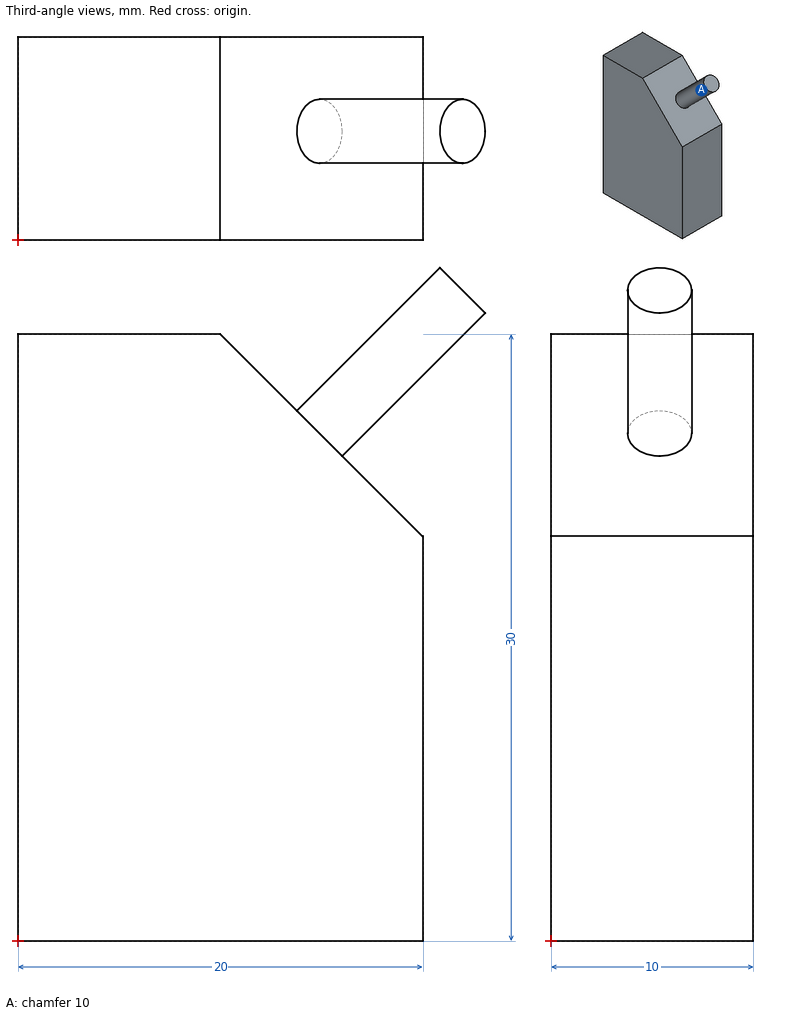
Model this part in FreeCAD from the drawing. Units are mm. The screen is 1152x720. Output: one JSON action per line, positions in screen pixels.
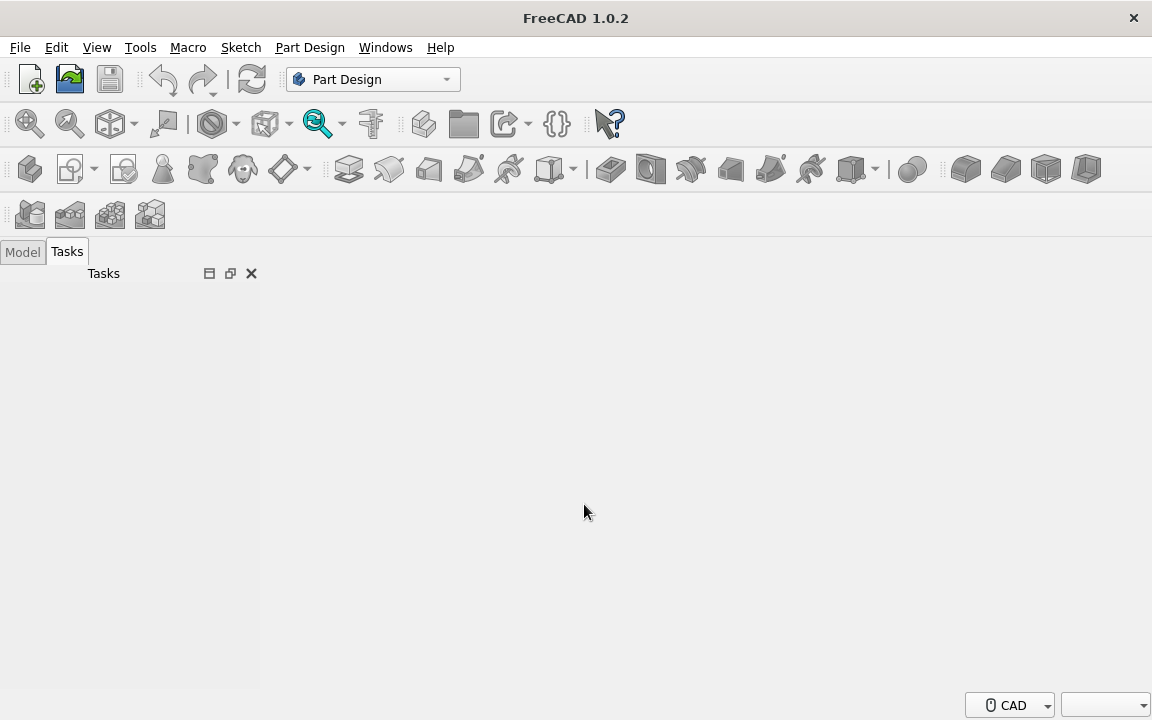
{"action": "key", "text": "ctrl+n"}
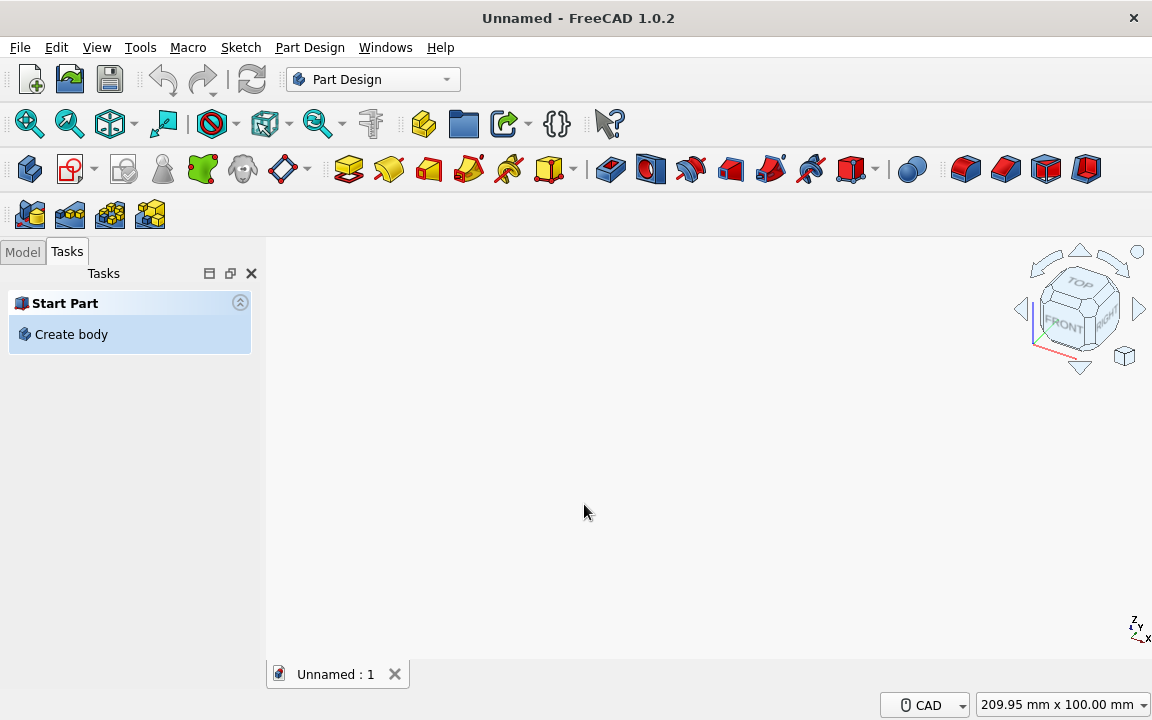
{"action": "left_click", "coordinate": [70, 170]}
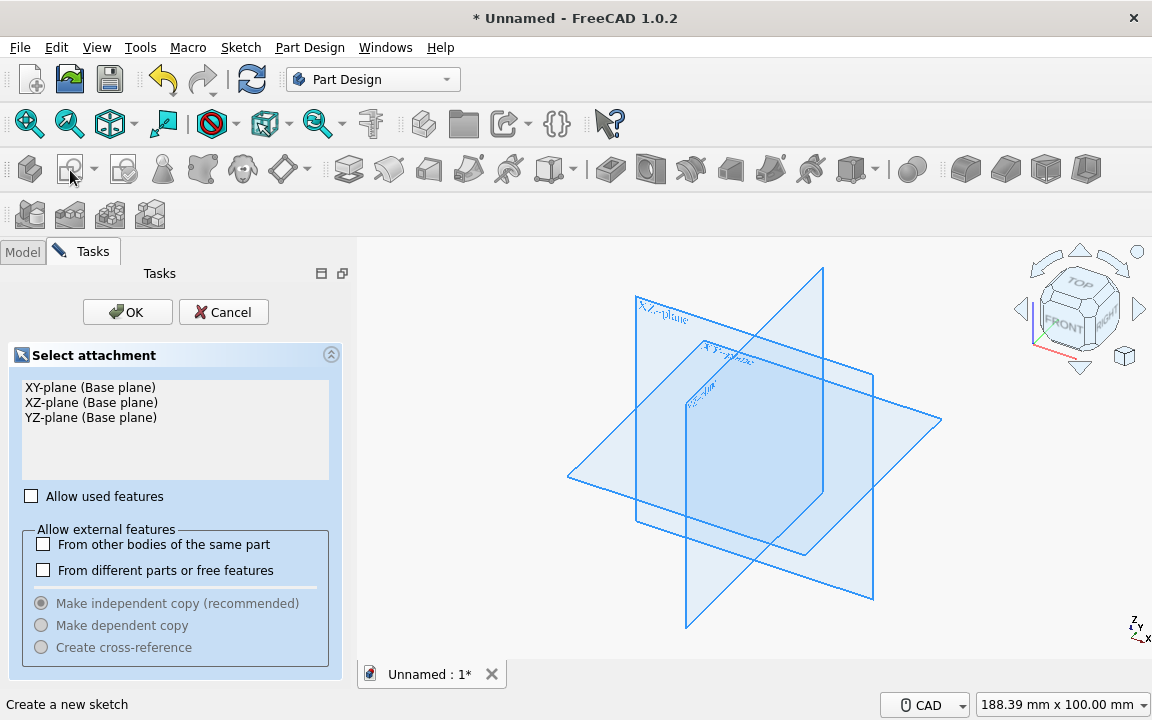
{"action": "left_click", "coordinate": [82, 402]}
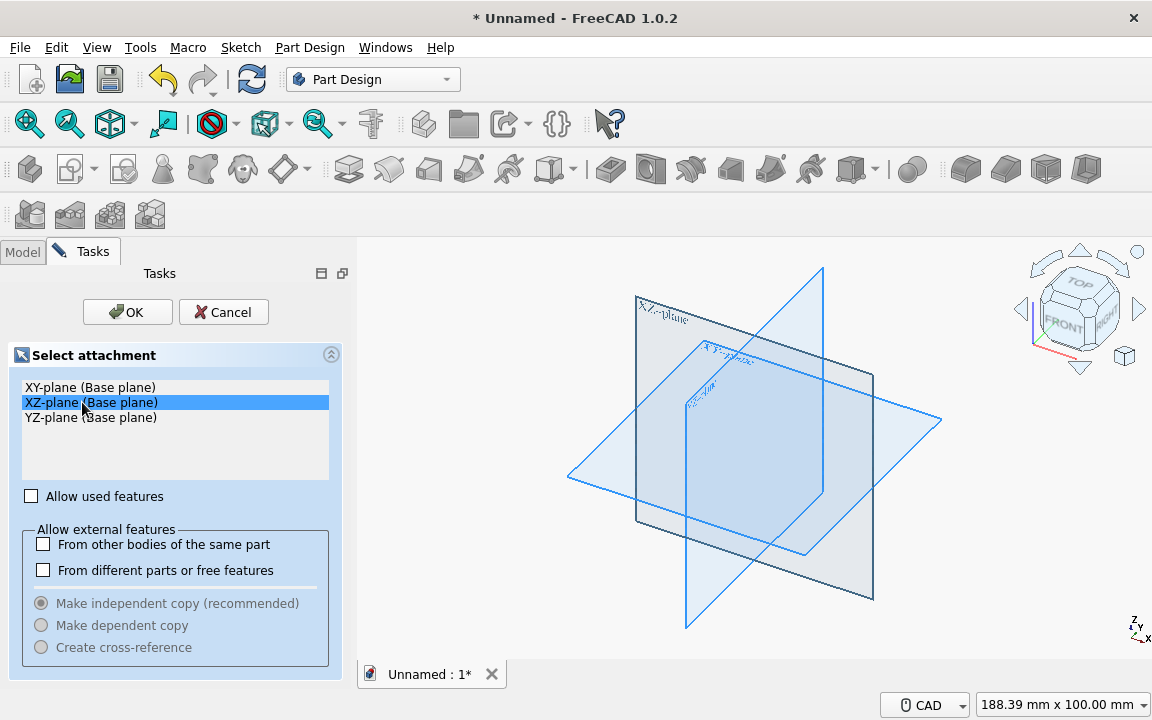
{"action": "left_click", "coordinate": [128, 312]}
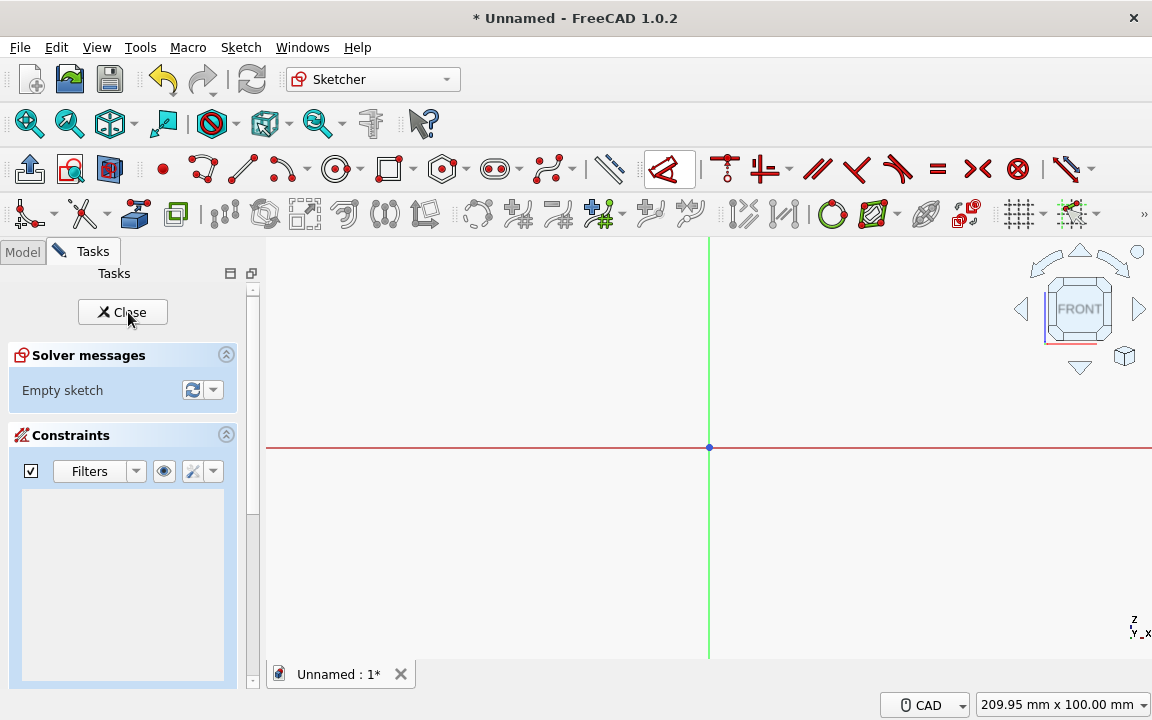
{"action": "scroll", "coordinate": [842, 333], "scroll_direction": "up", "scroll_amount": 4}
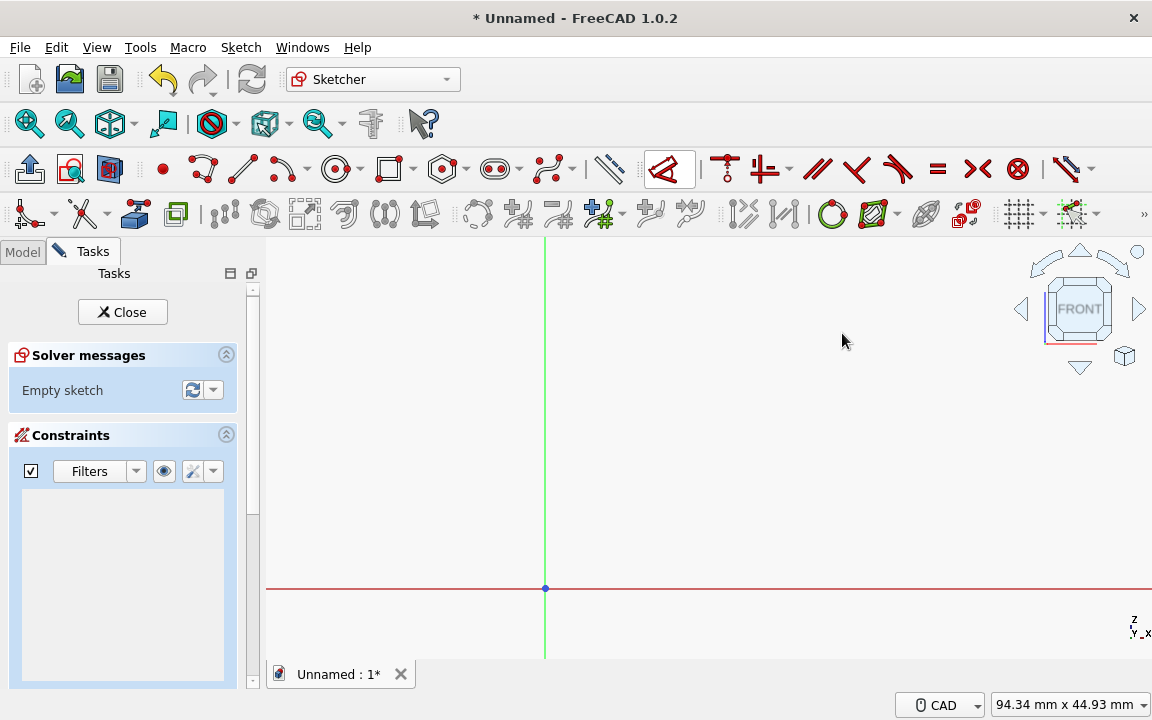
{"action": "key", "text": "g r"}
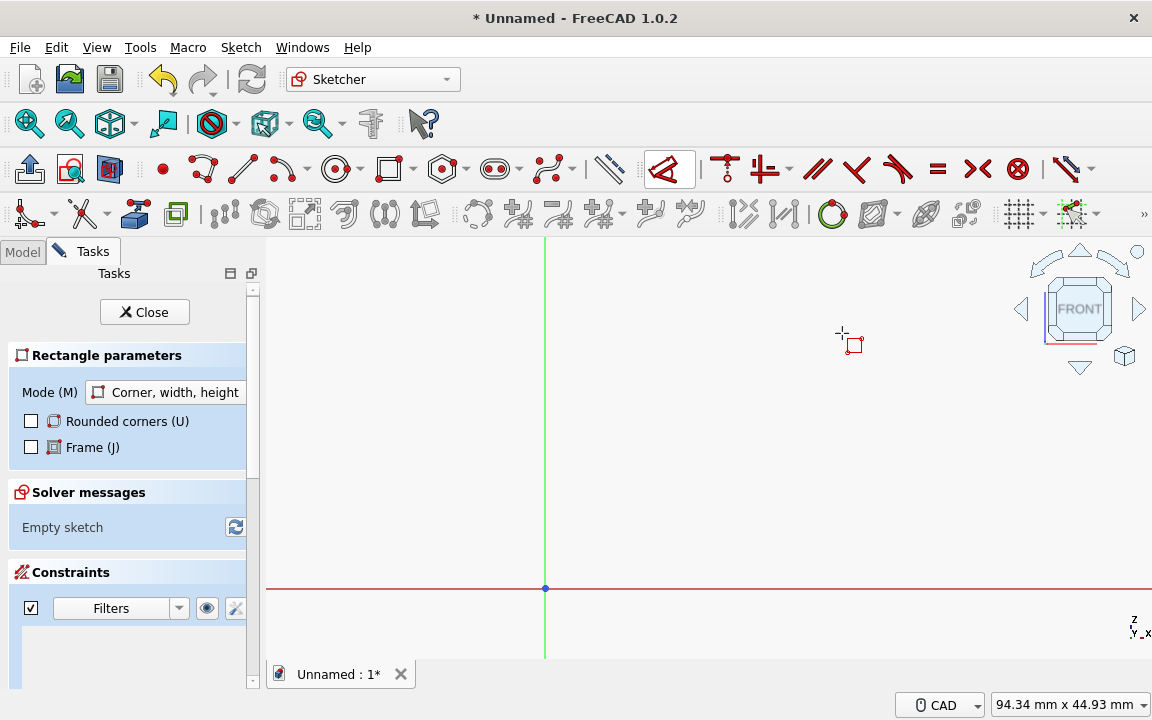
{"action": "left_click", "coordinate": [545, 589]}
{"action": "mouse_move", "coordinate": [733, 307]}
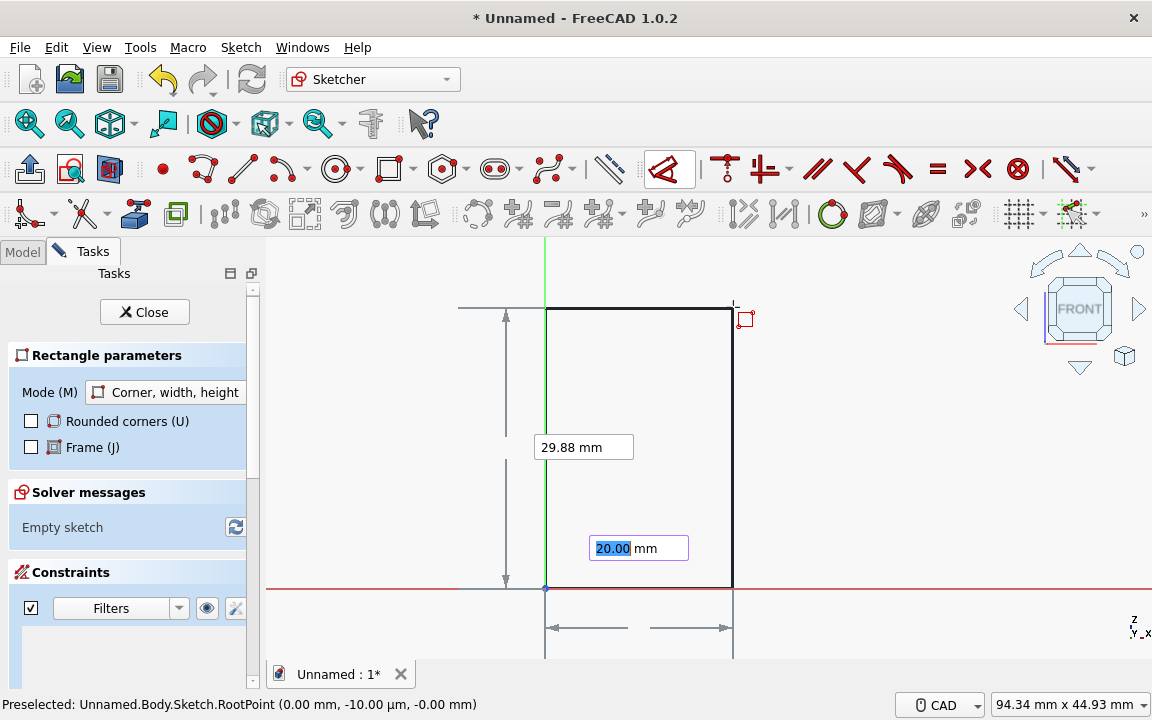
{"action": "type", "text": "20"}
{"action": "key", "text": "Tab"}
{"action": "type", "text": "30"}
{"action": "key", "text": "Return"}
{"action": "key", "text": "Escape"}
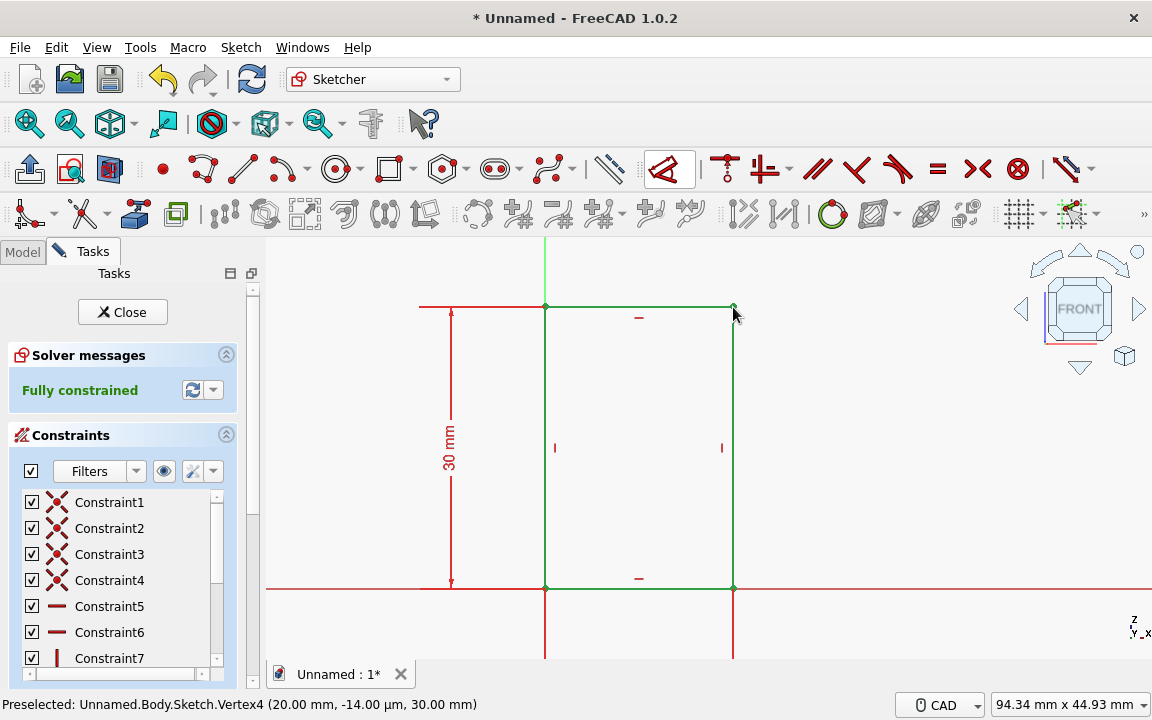
{"action": "left_click", "coordinate": [123, 312]}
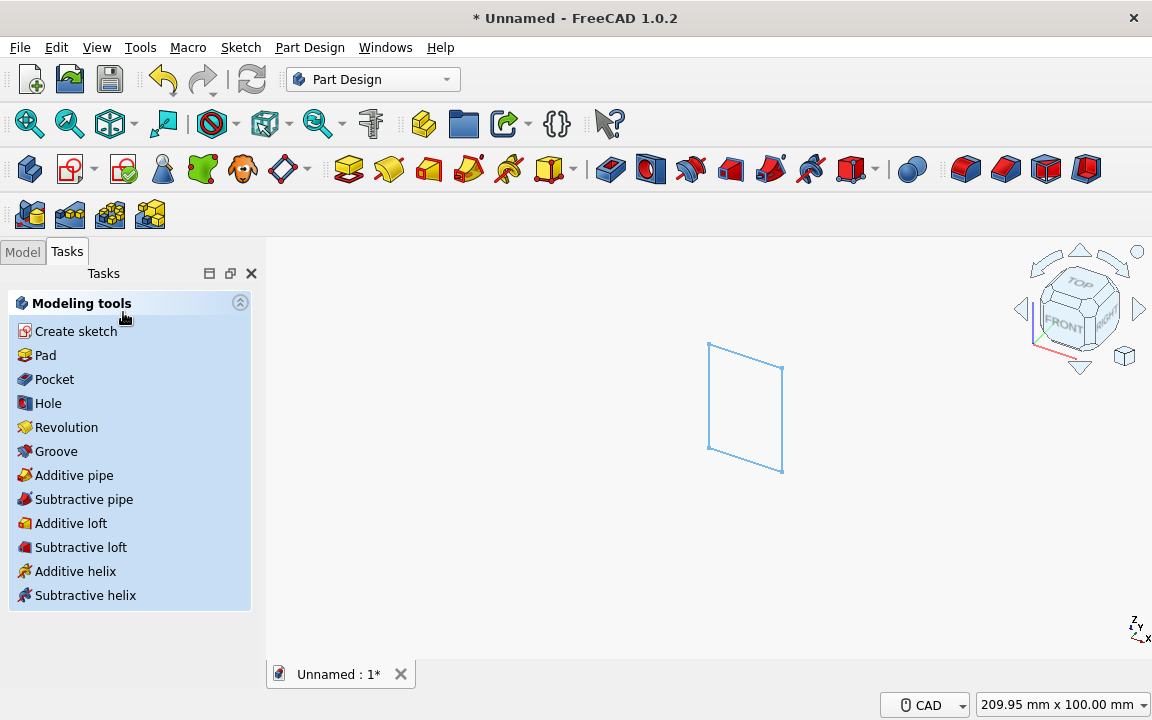
{"action": "left_click", "coordinate": [350, 170]}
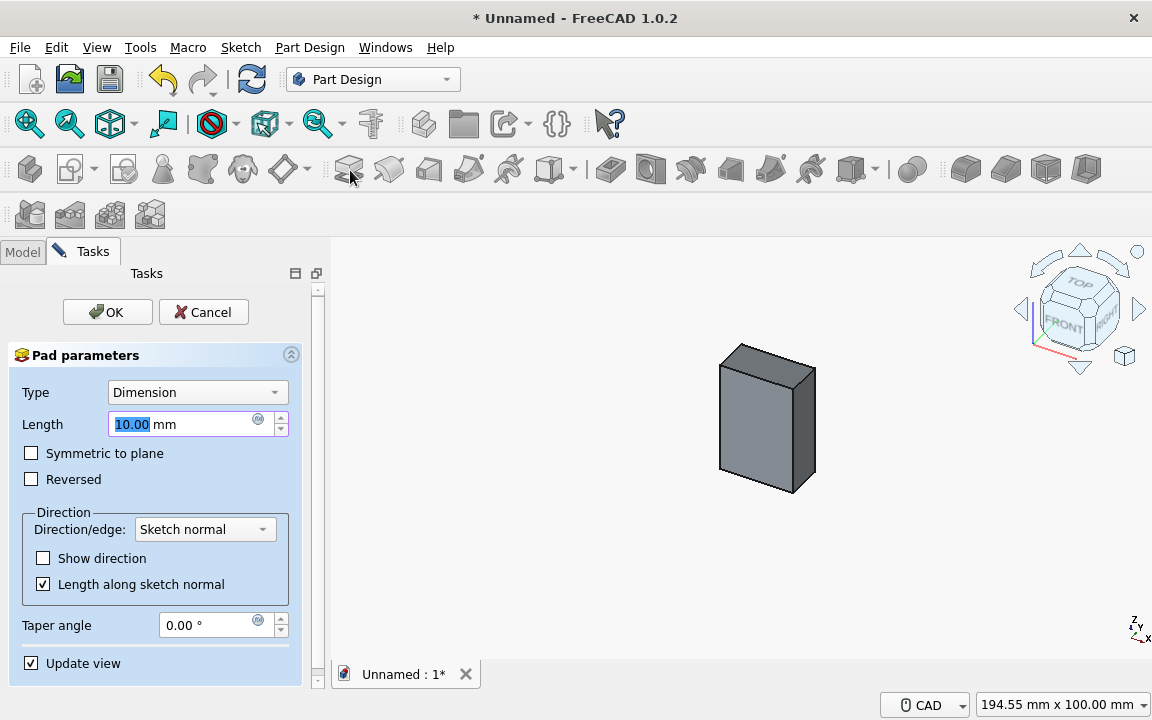
{"action": "type", "text": "10"}
{"action": "key", "text": "Tab"}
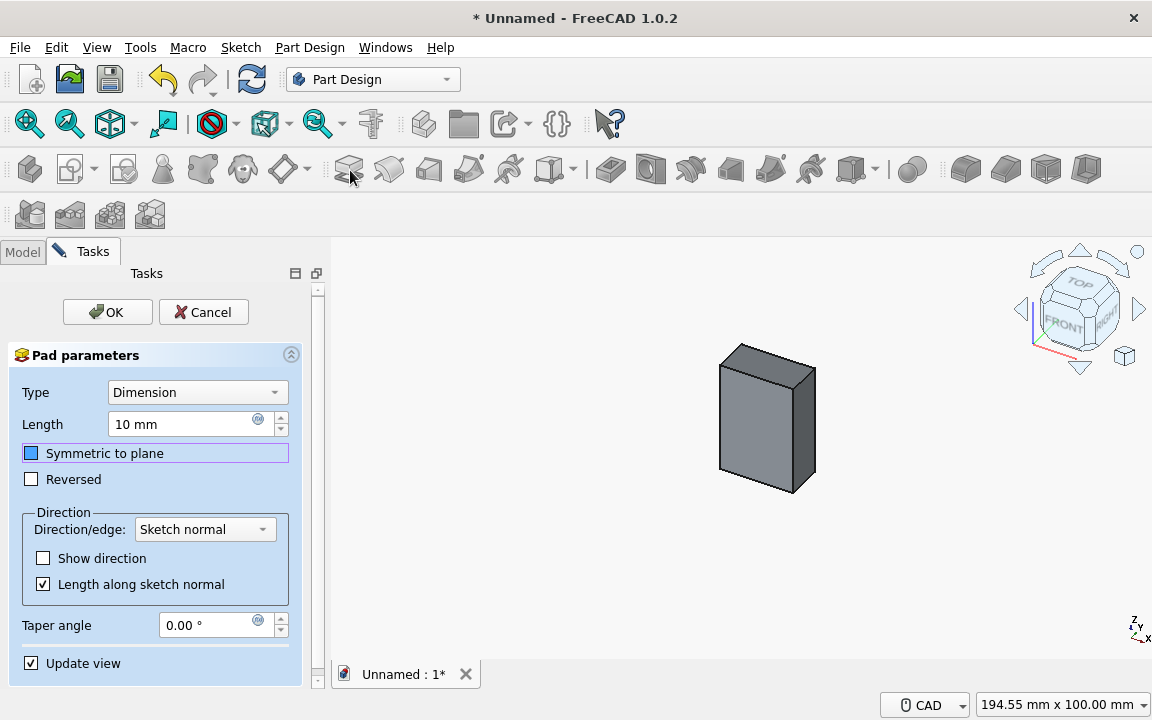
{"action": "left_click", "coordinate": [30, 479]}